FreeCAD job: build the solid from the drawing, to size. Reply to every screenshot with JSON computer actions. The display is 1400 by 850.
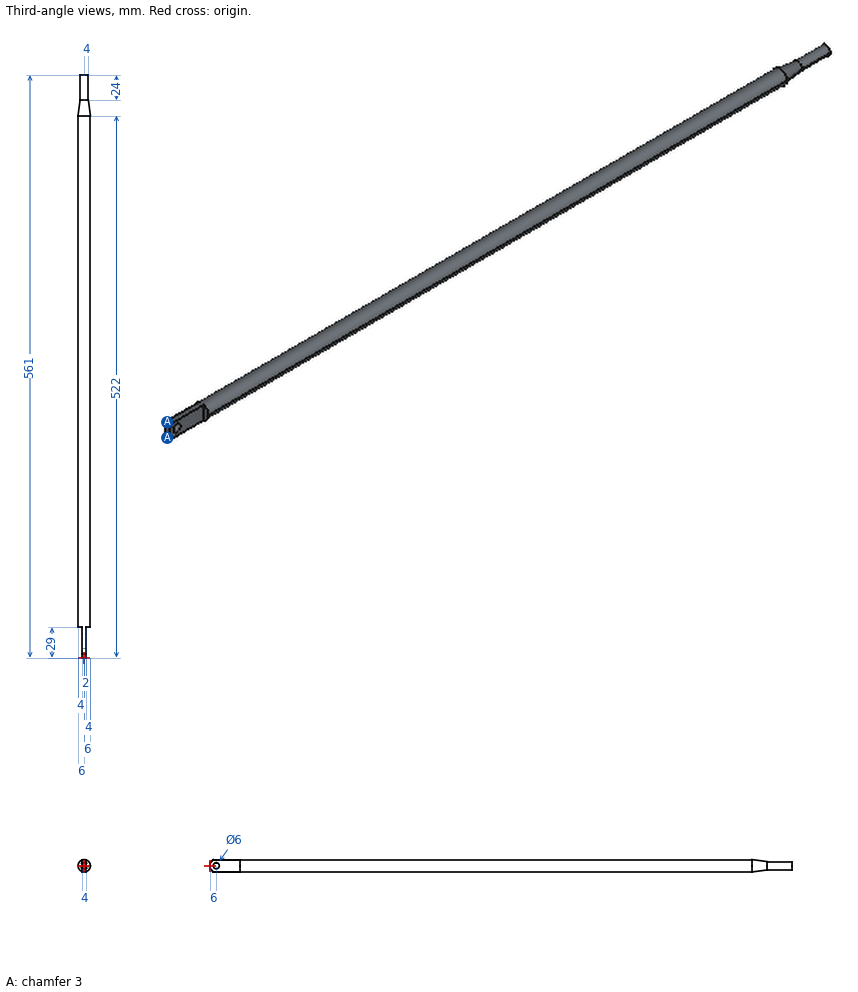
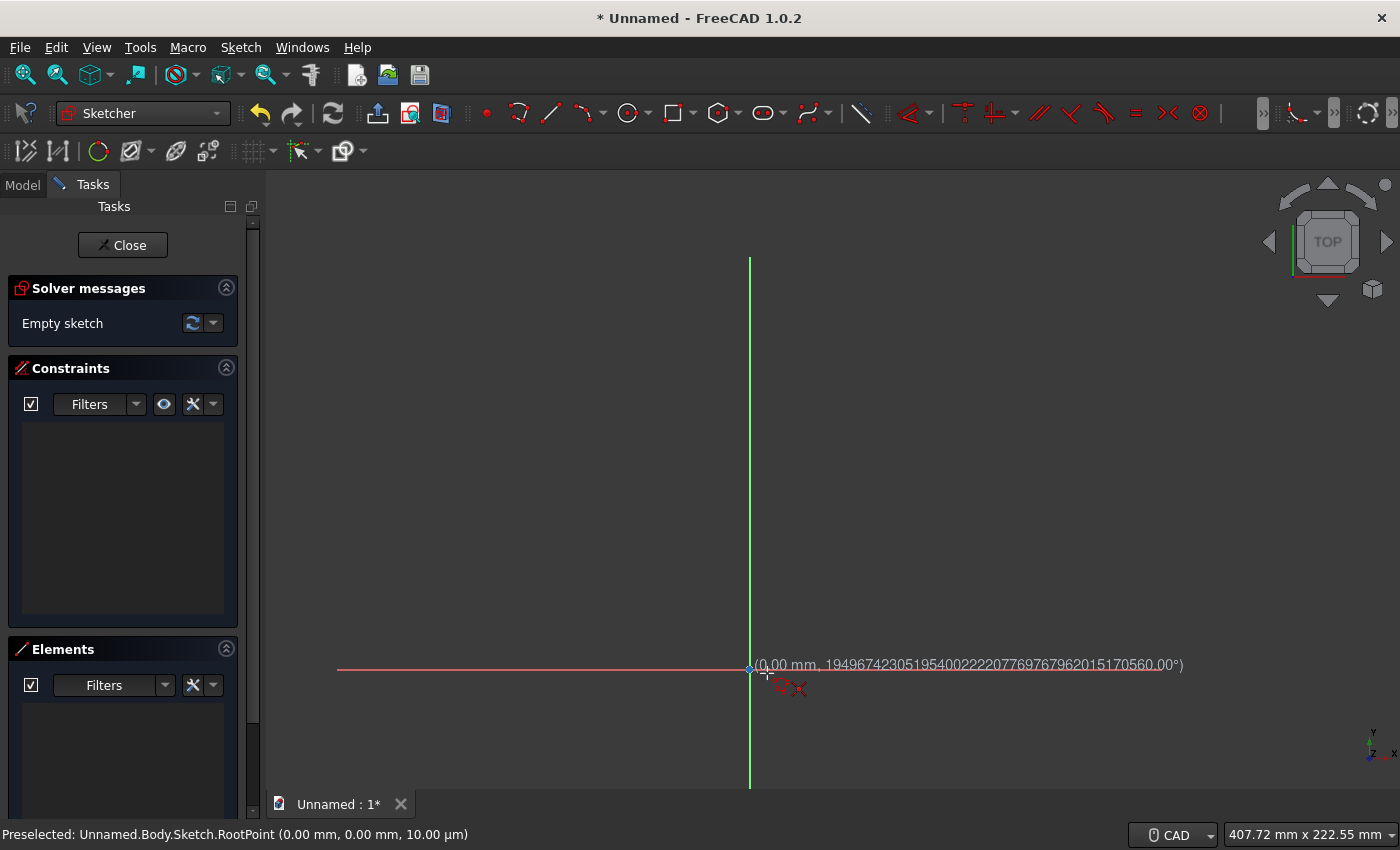
{"action": "left_click", "coordinate": [767, 661]}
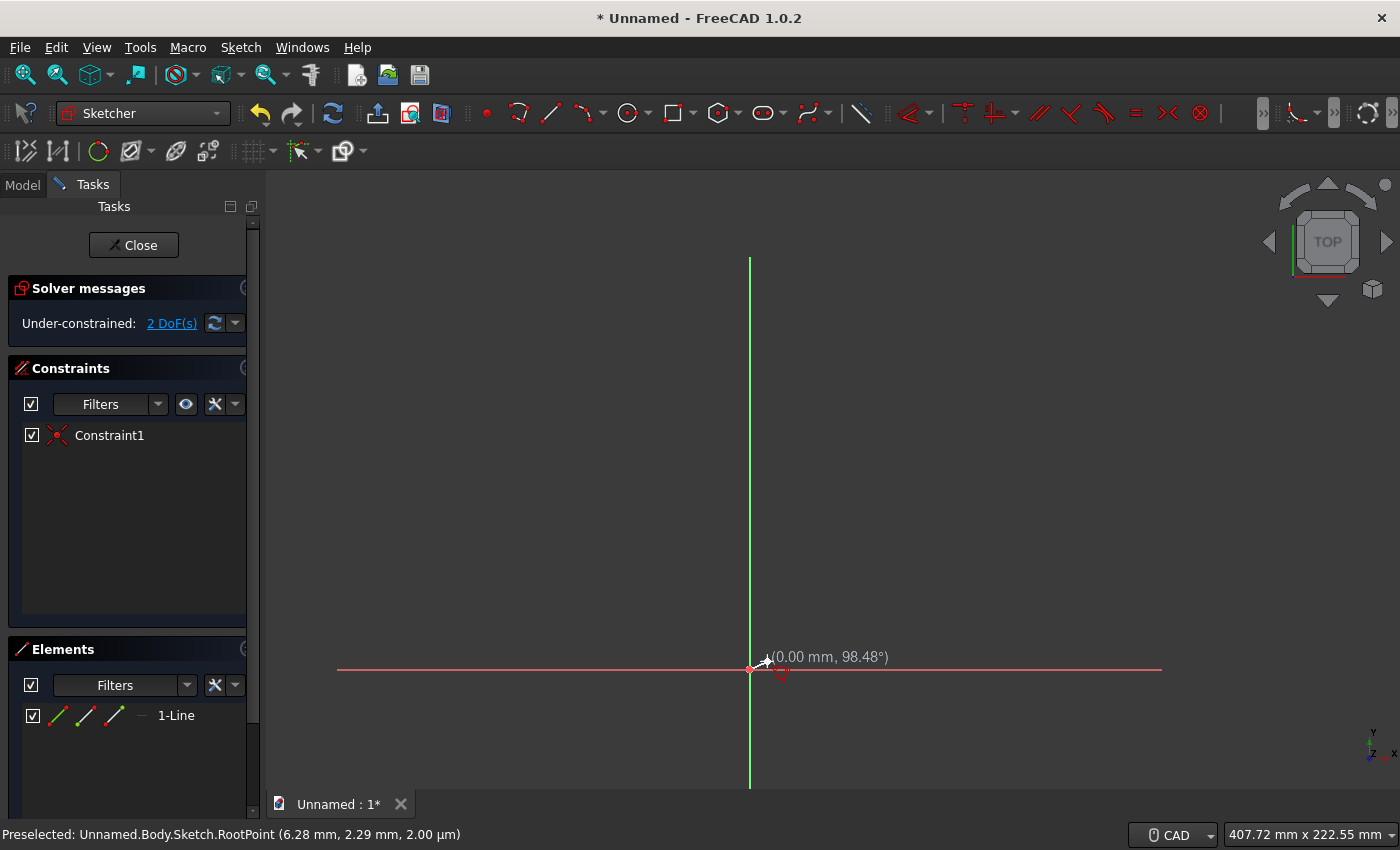
{"action": "scroll", "coordinate": [767, 673], "scroll_direction": "down", "scroll_amount": 7}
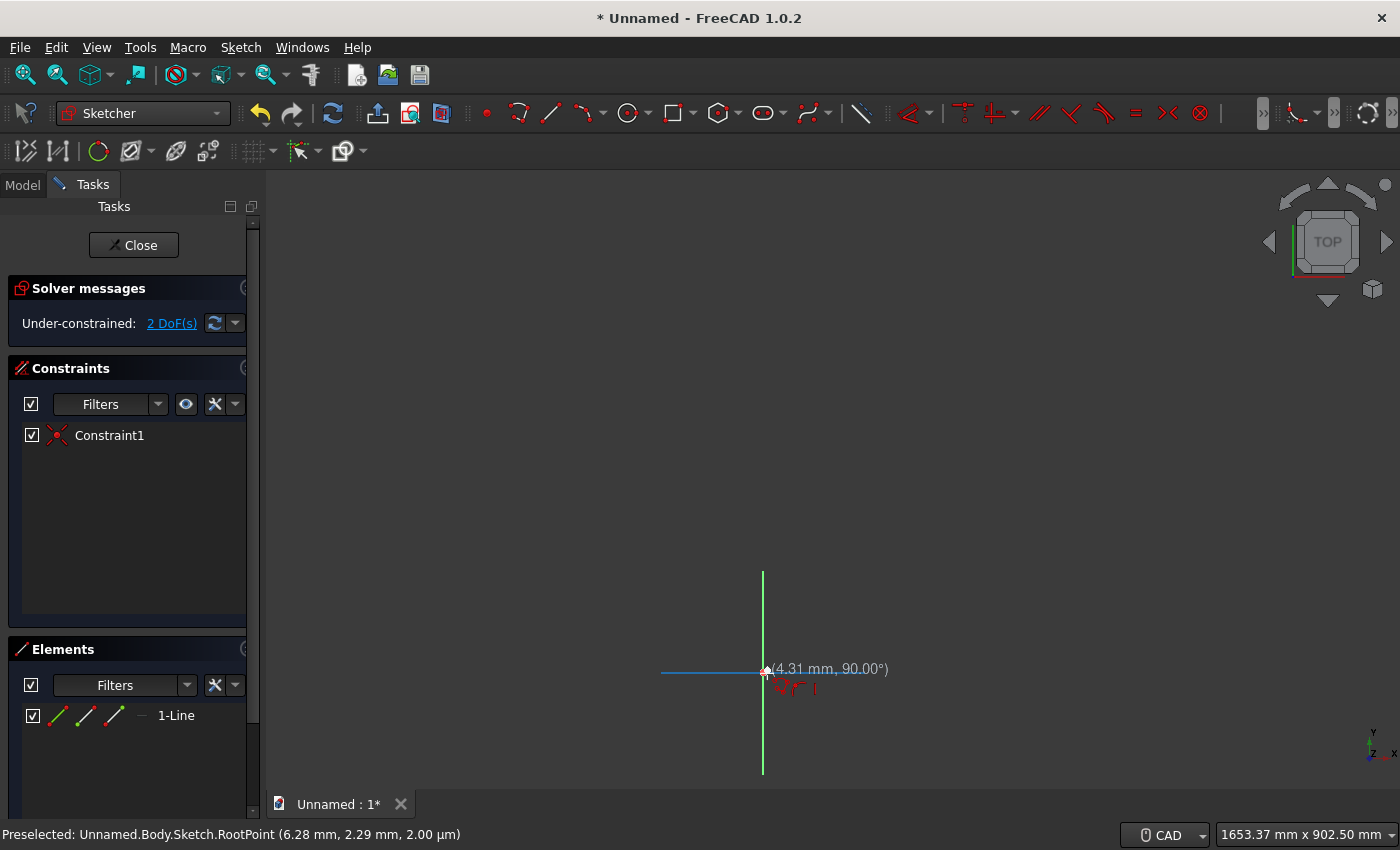
{"action": "scroll", "coordinate": [767, 315], "scroll_direction": "up", "scroll_amount": 7}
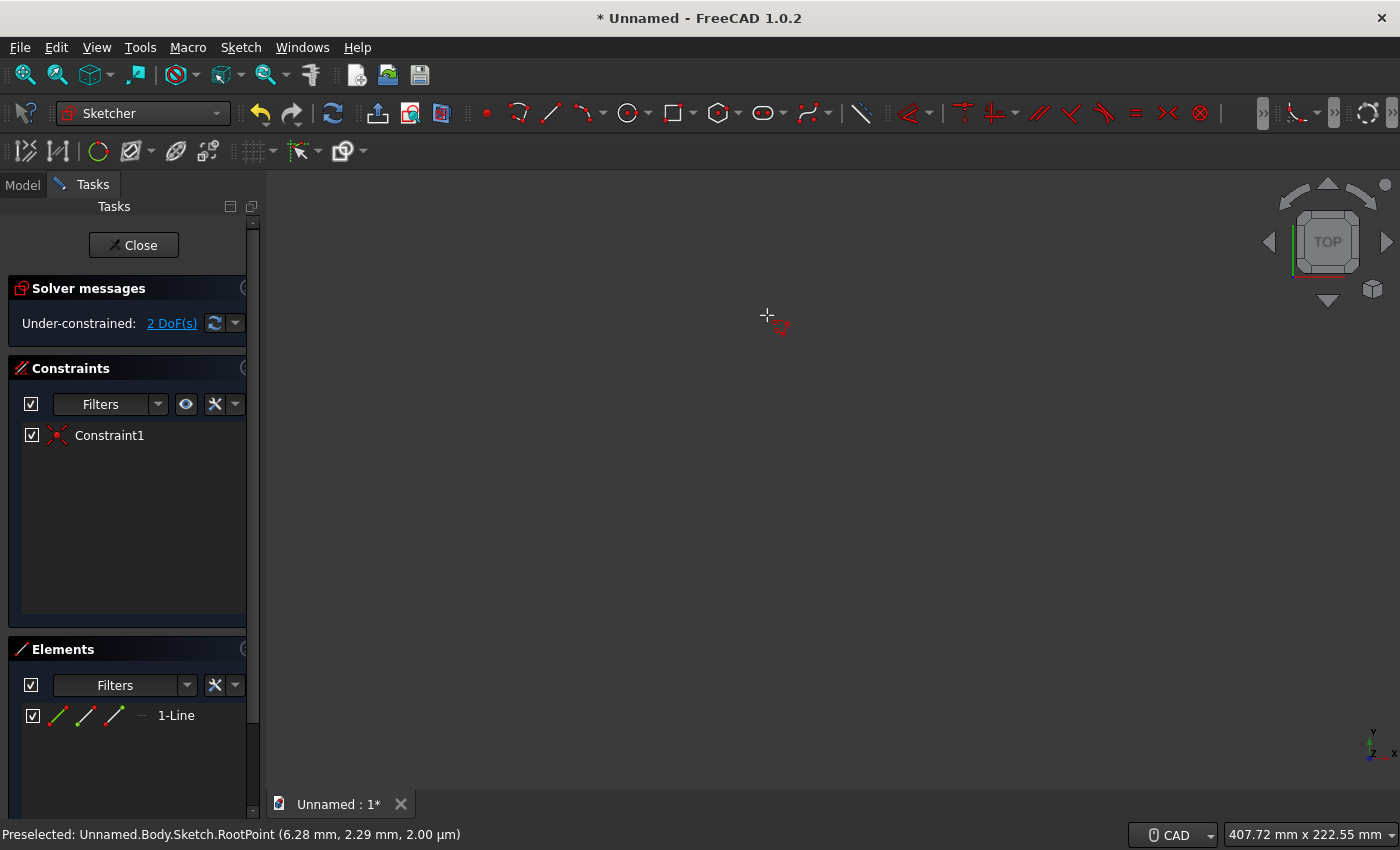
{"action": "left_click", "coordinate": [767, 313]}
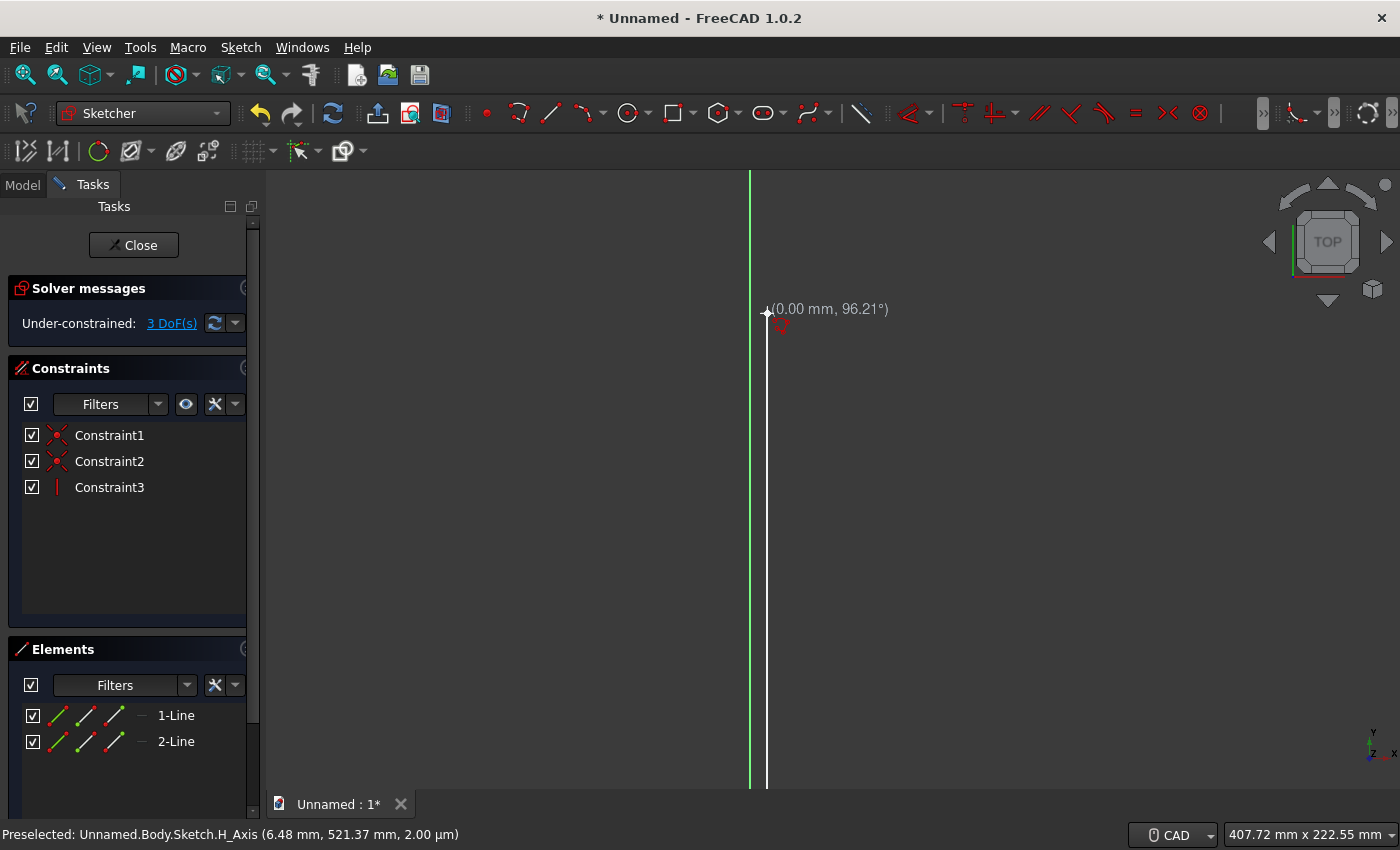
{"action": "scroll", "coordinate": [761, 272], "scroll_direction": "up", "scroll_amount": 2}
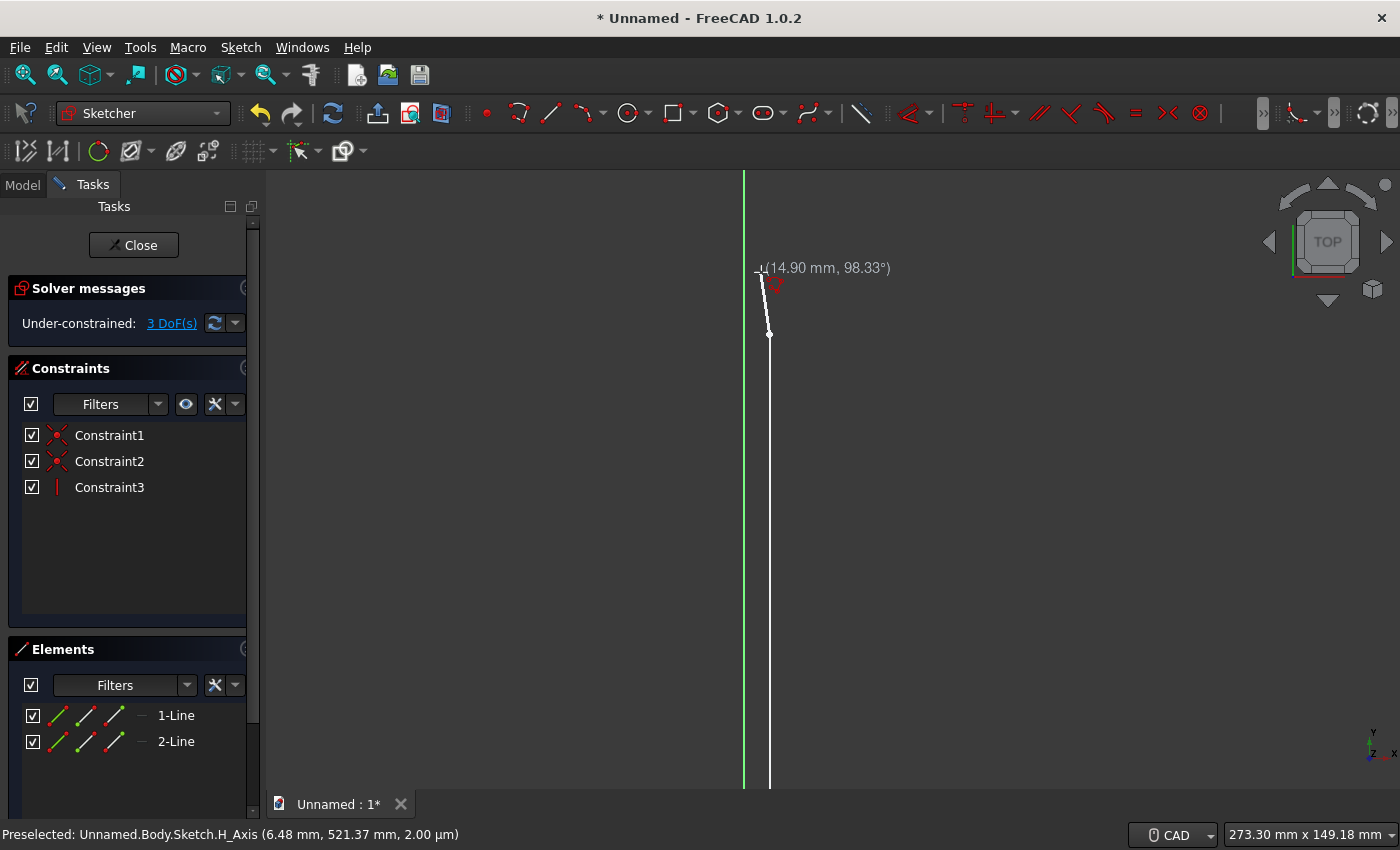
{"action": "left_click", "coordinate": [761, 271]}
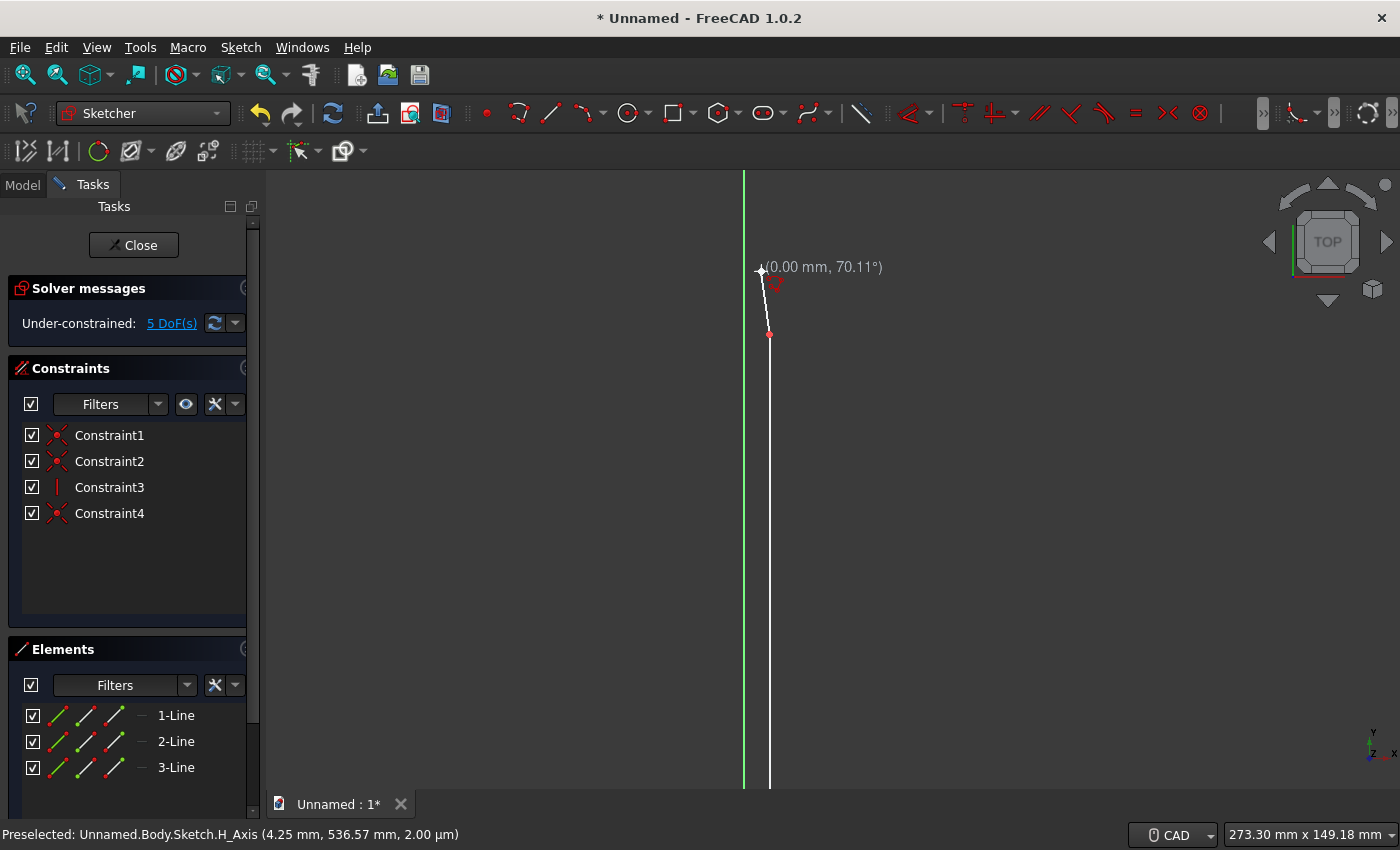
{"action": "scroll", "coordinate": [766, 310], "scroll_direction": "down", "scroll_amount": 9}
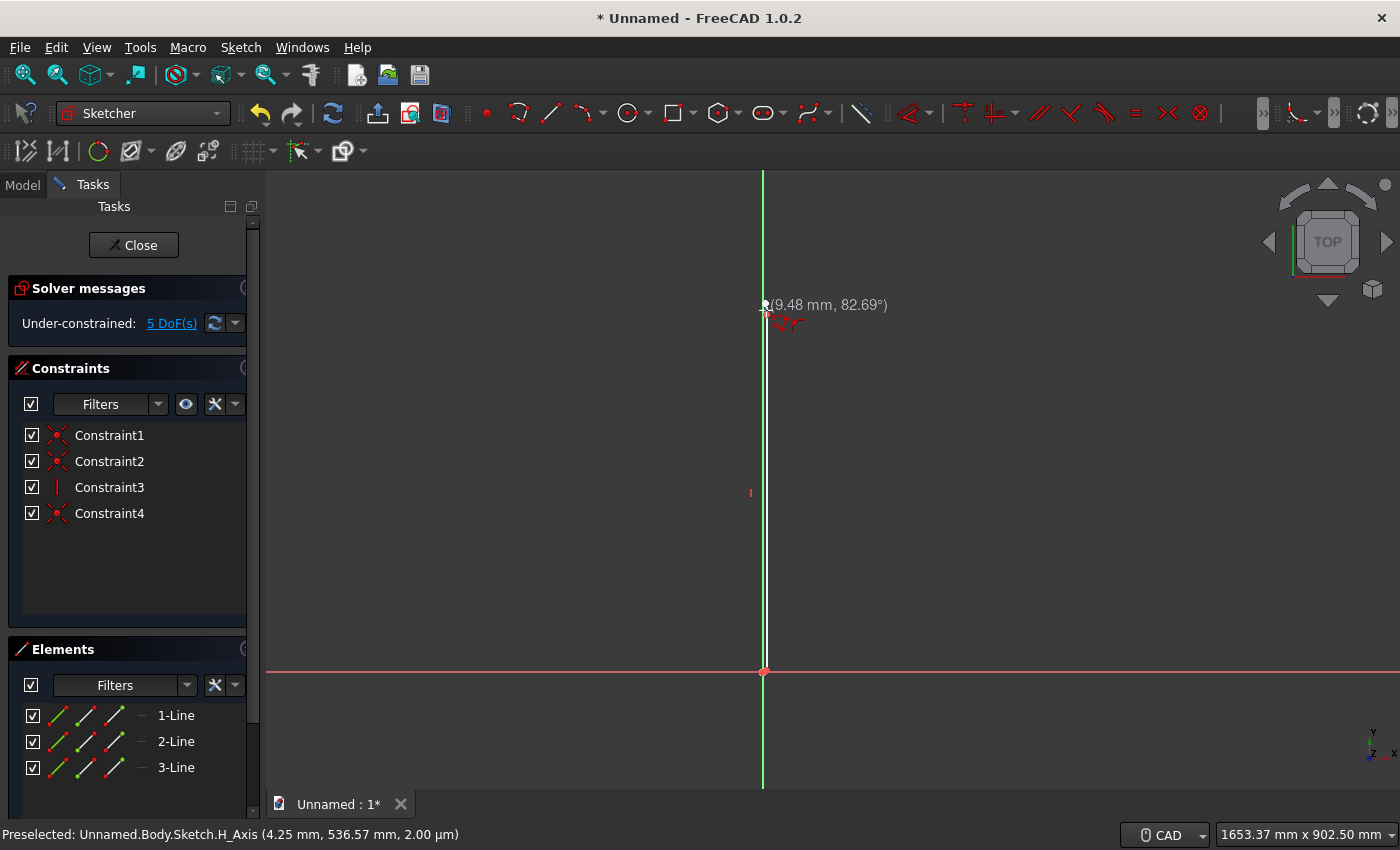
{"action": "scroll", "coordinate": [766, 287], "scroll_direction": "up", "scroll_amount": 9}